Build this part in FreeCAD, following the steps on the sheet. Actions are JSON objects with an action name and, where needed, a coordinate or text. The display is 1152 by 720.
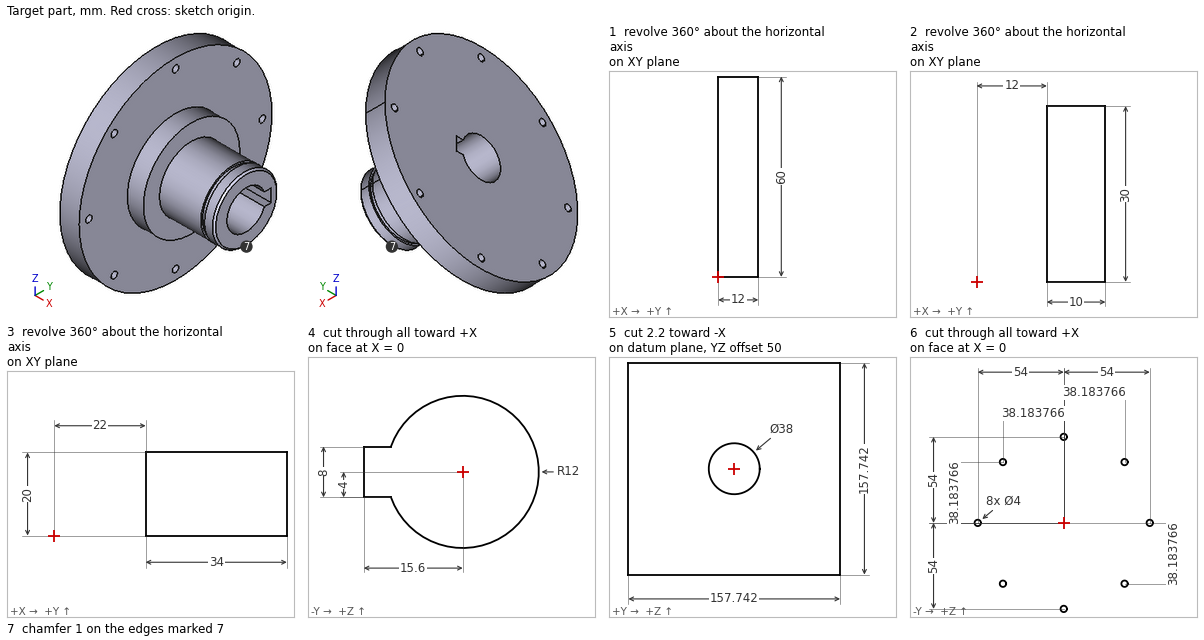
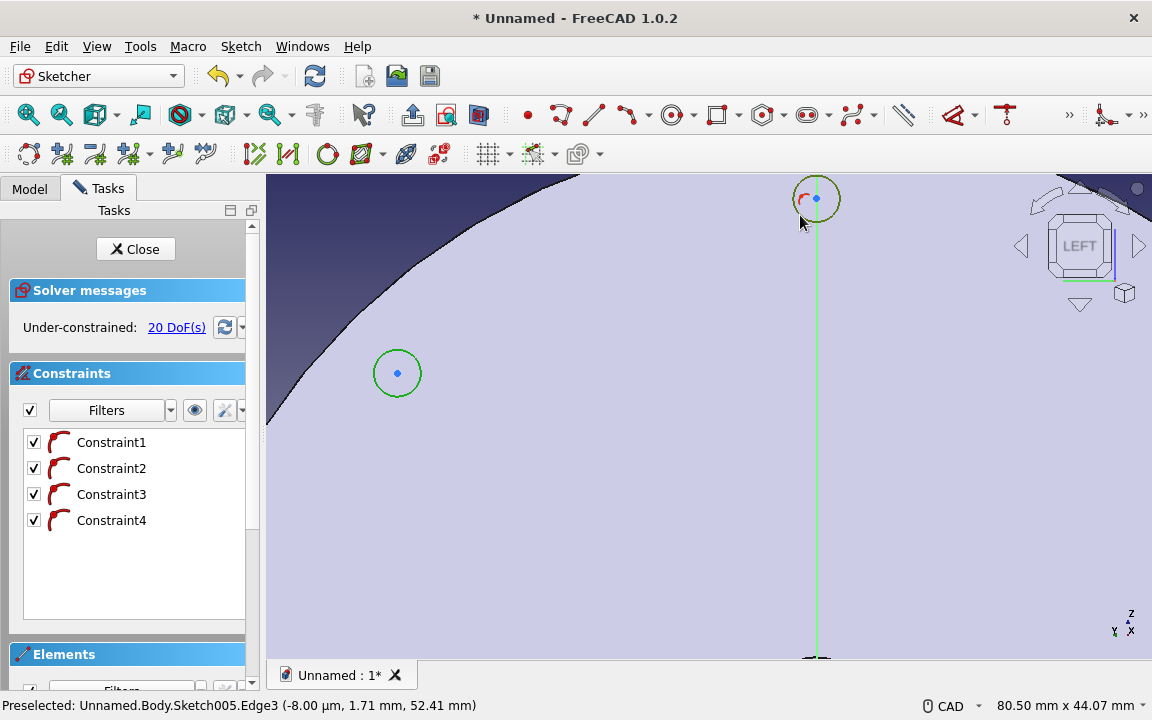
{"action": "scroll", "coordinate": [583, 294], "scroll_direction": "down", "scroll_amount": 7}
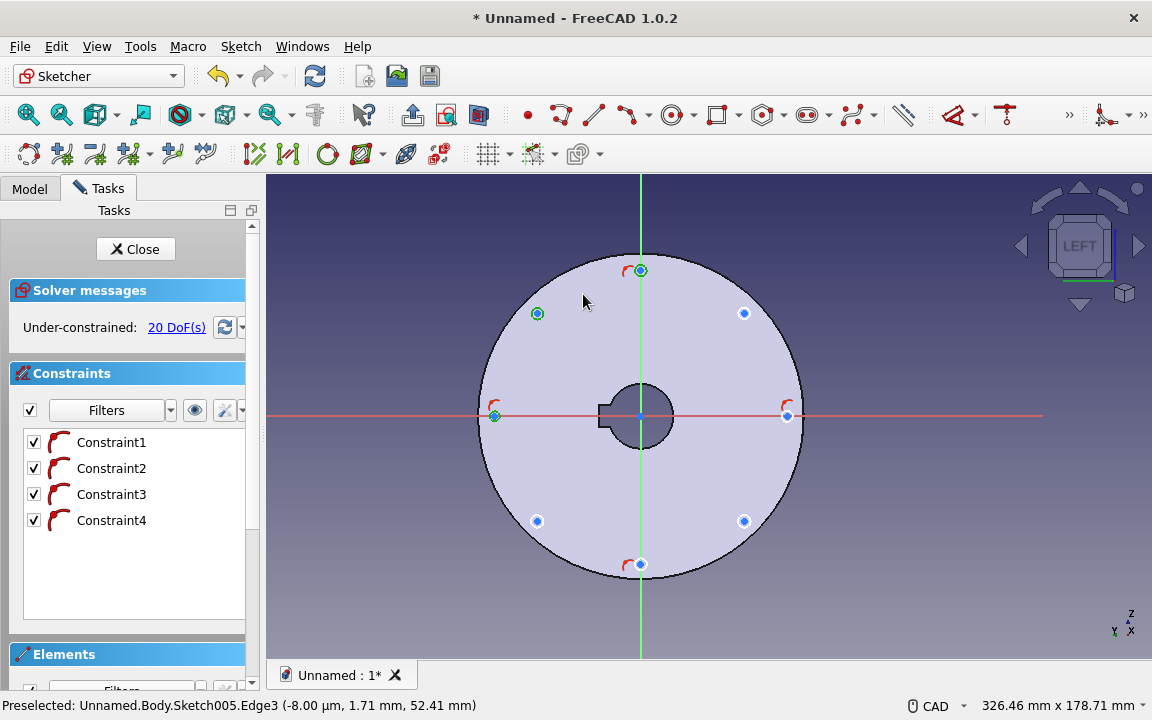
{"action": "scroll", "coordinate": [748, 309], "scroll_direction": "up", "scroll_amount": 5}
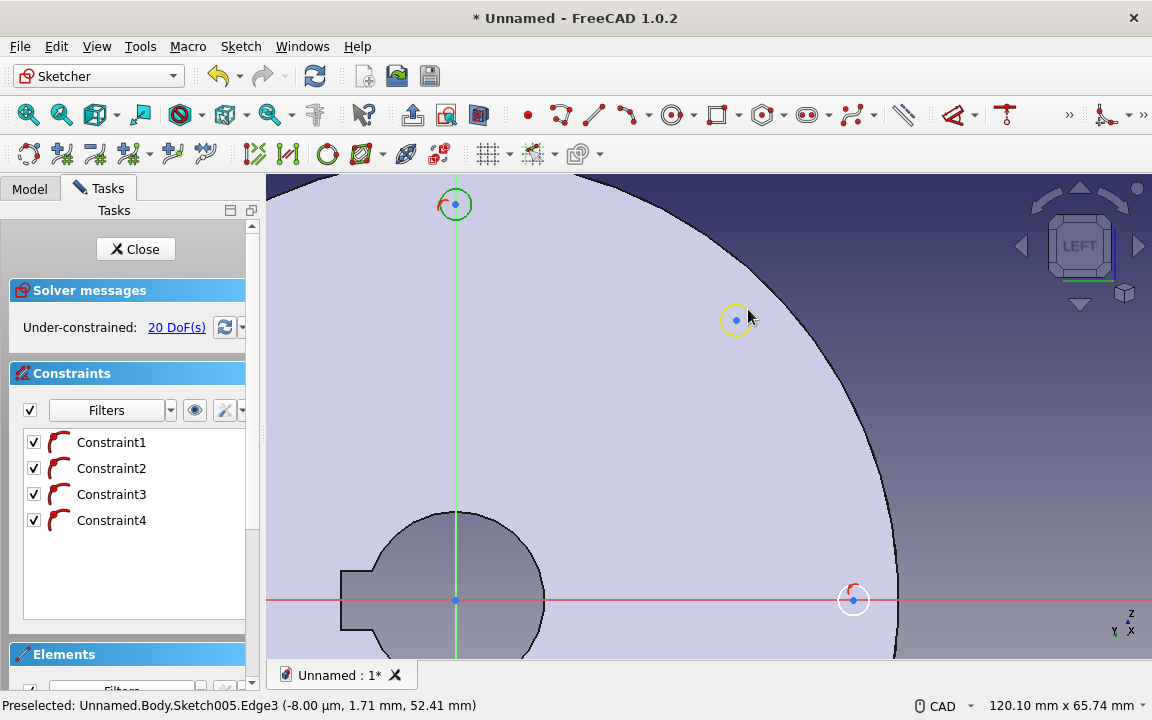
{"action": "left_click", "coordinate": [748, 309]}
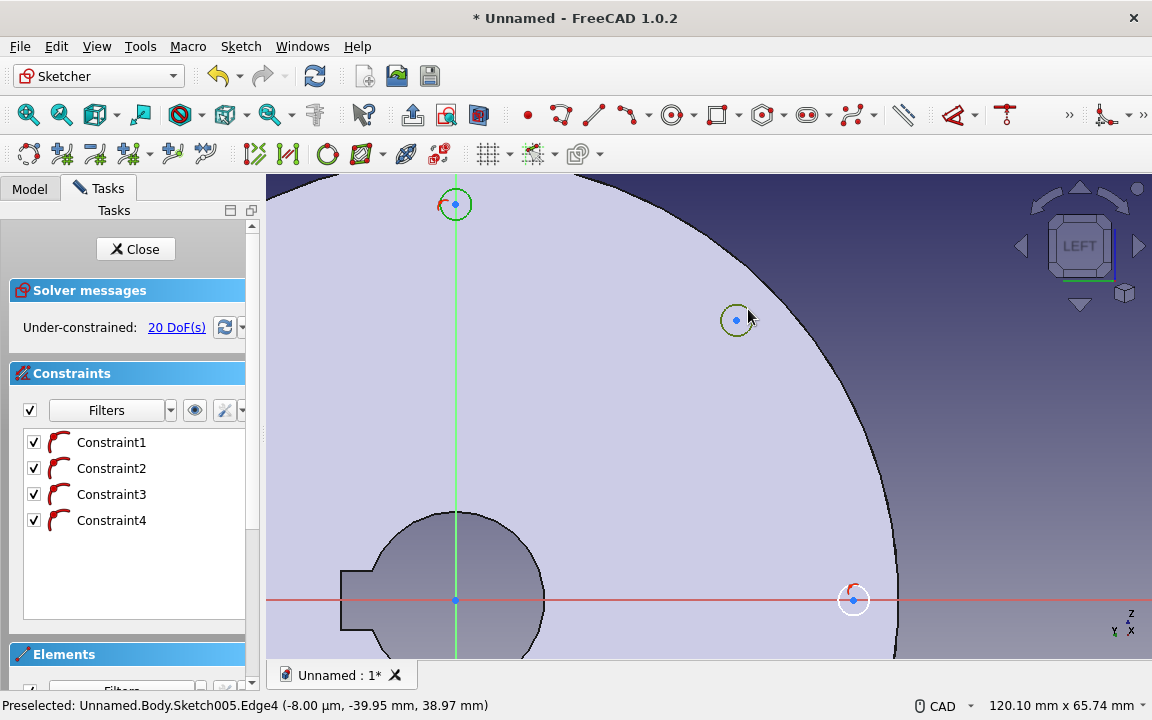
{"action": "scroll", "coordinate": [864, 589], "scroll_direction": "up", "scroll_amount": 2}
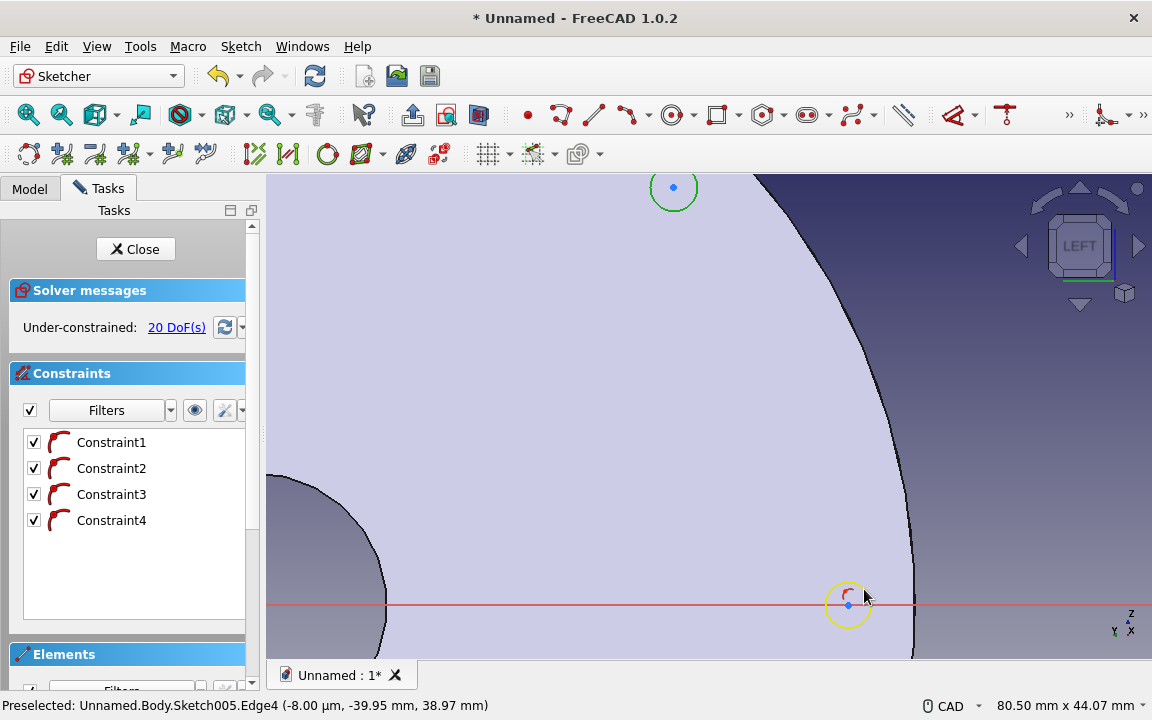
{"action": "left_click", "coordinate": [864, 589]}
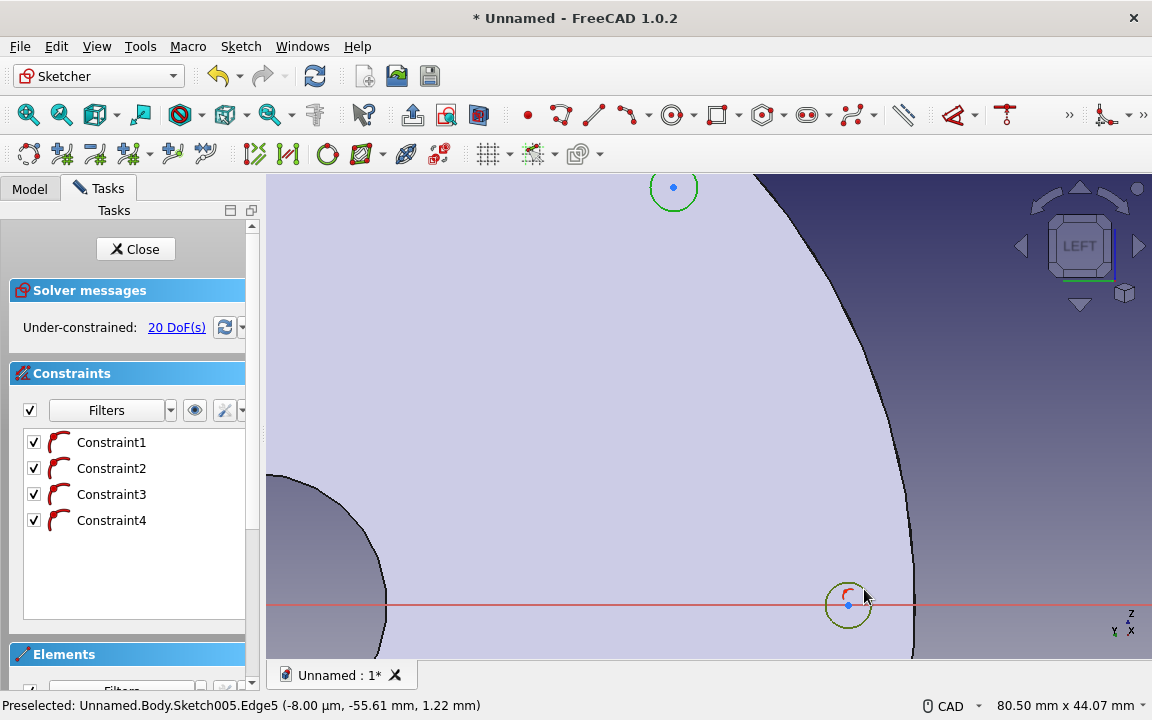
{"action": "scroll", "coordinate": [767, 355], "scroll_direction": "down", "scroll_amount": 7}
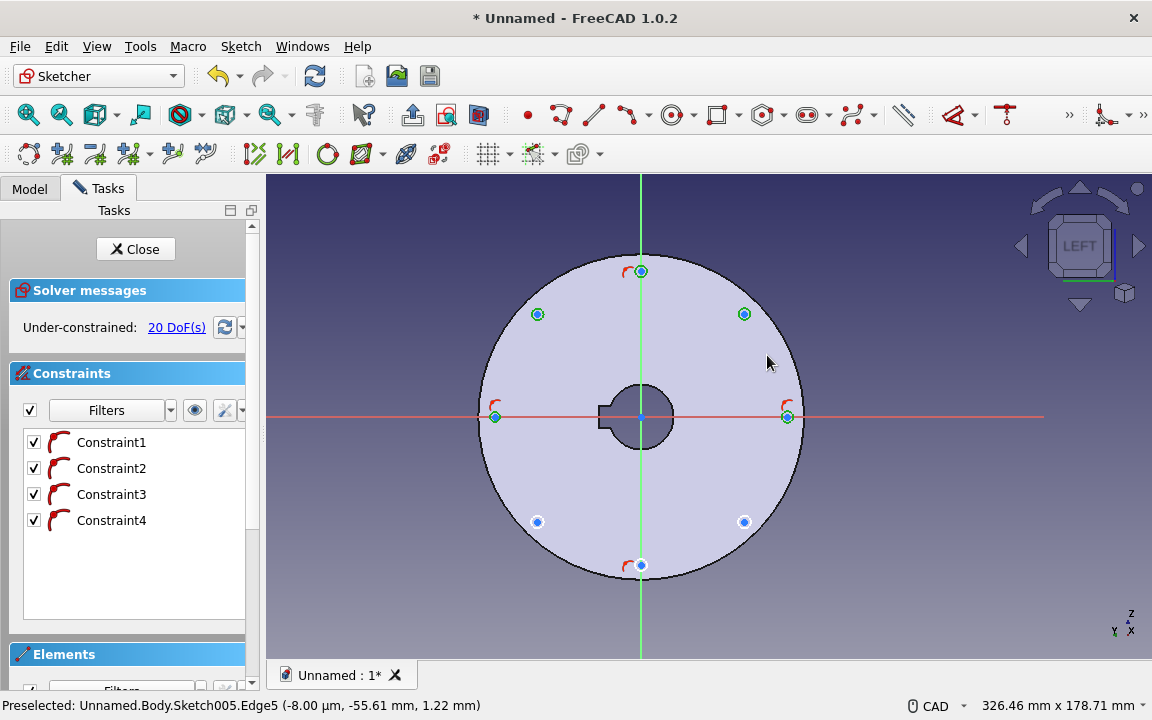
{"action": "scroll", "coordinate": [749, 518], "scroll_direction": "up", "scroll_amount": 4}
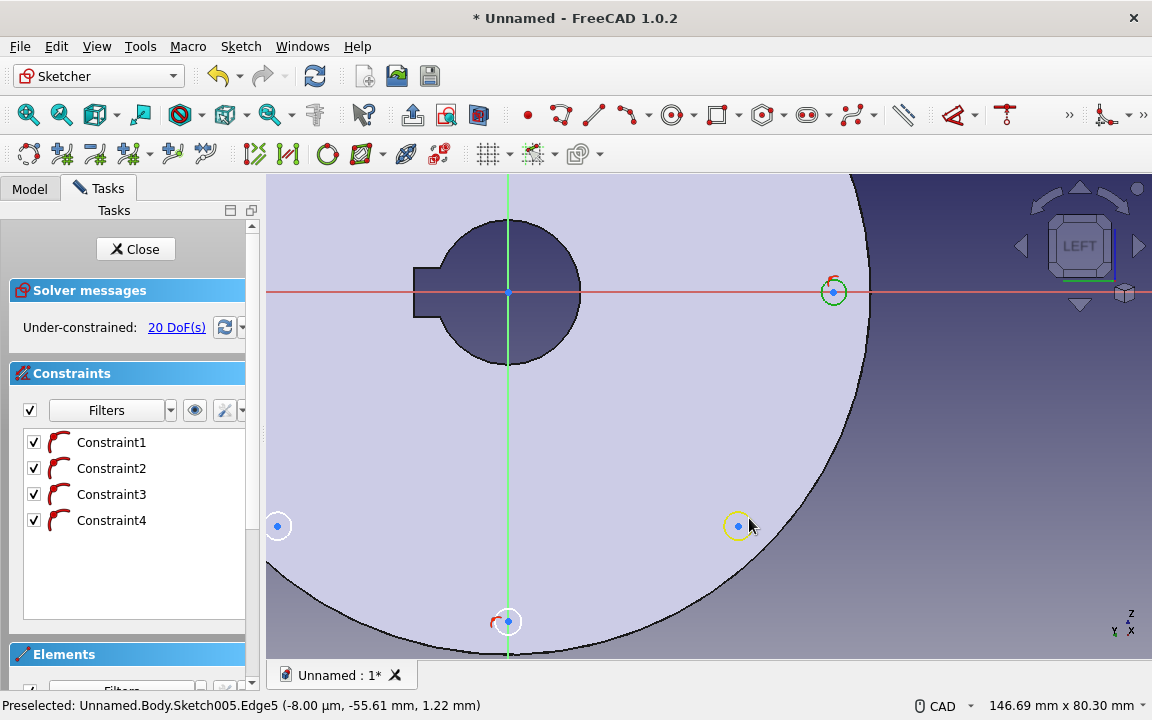
{"action": "left_click", "coordinate": [748, 516]}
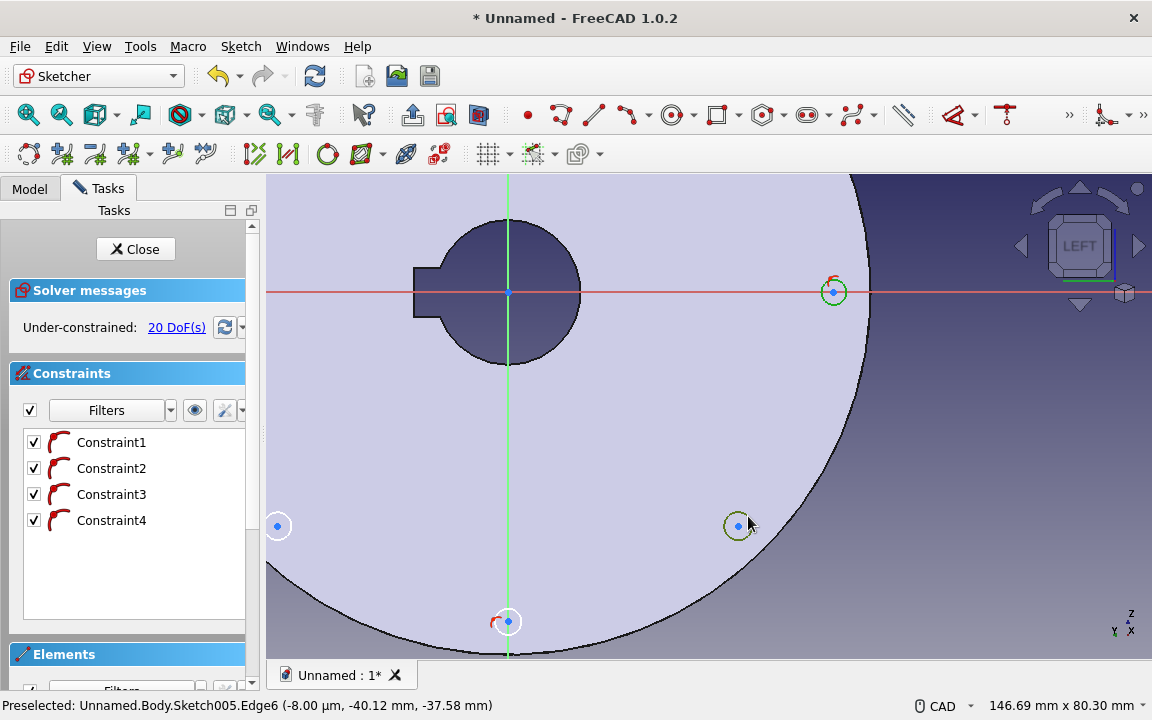
{"action": "scroll", "coordinate": [517, 613], "scroll_direction": "up", "scroll_amount": 2}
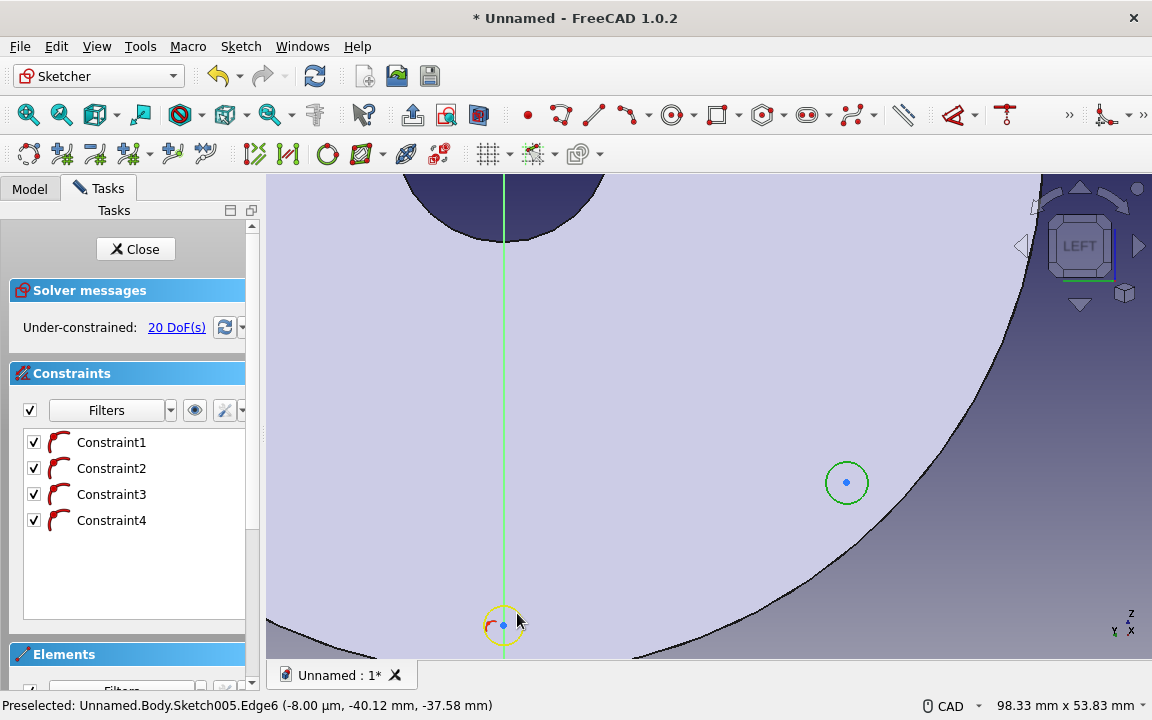
{"action": "left_click", "coordinate": [518, 612]}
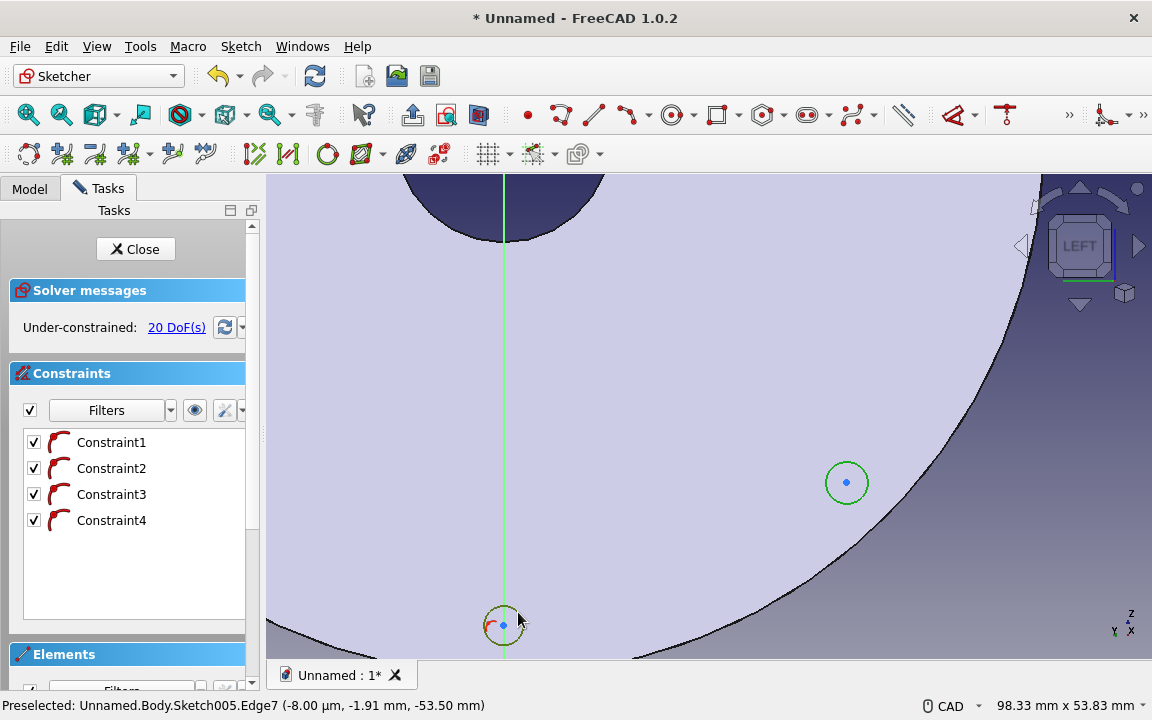
{"action": "scroll", "coordinate": [699, 538], "scroll_direction": "down", "scroll_amount": 6}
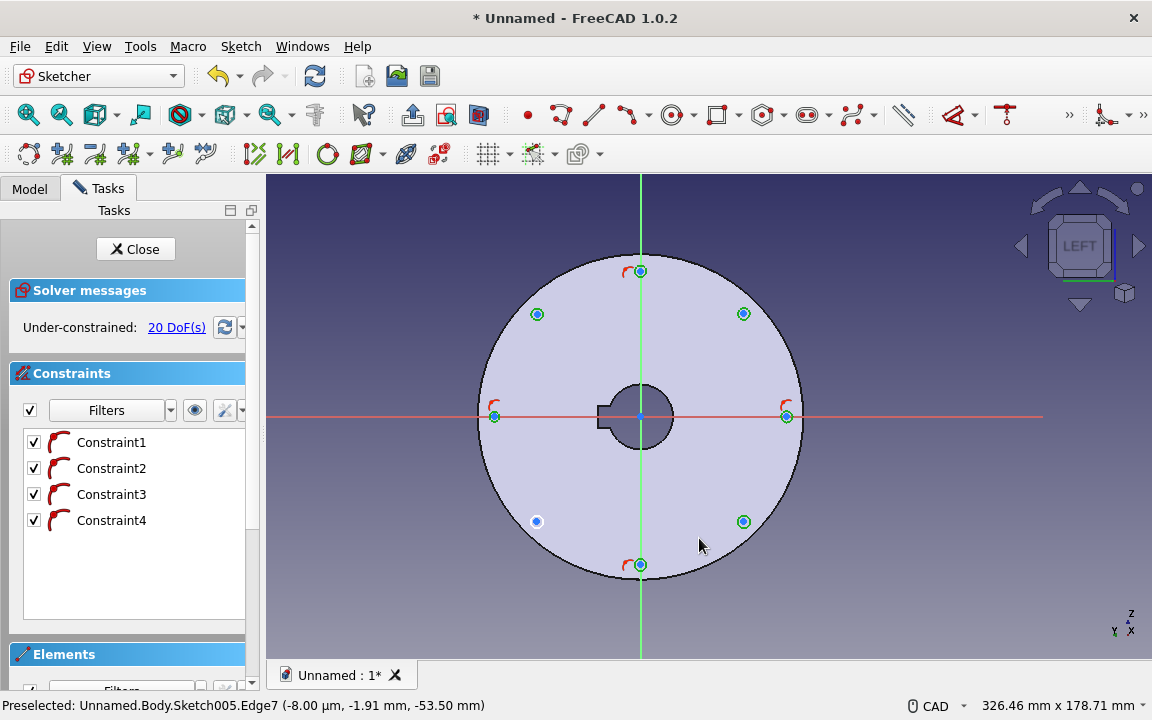
{"action": "scroll", "coordinate": [541, 518], "scroll_direction": "up", "scroll_amount": 5}